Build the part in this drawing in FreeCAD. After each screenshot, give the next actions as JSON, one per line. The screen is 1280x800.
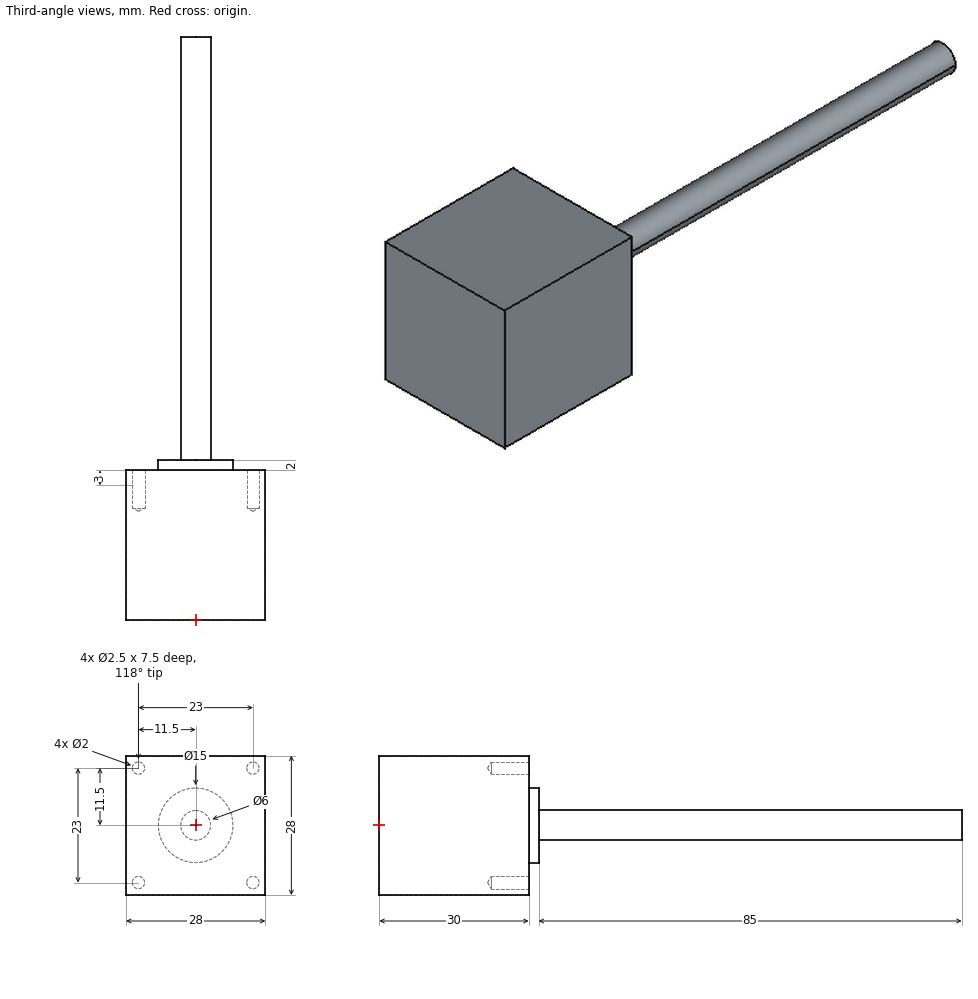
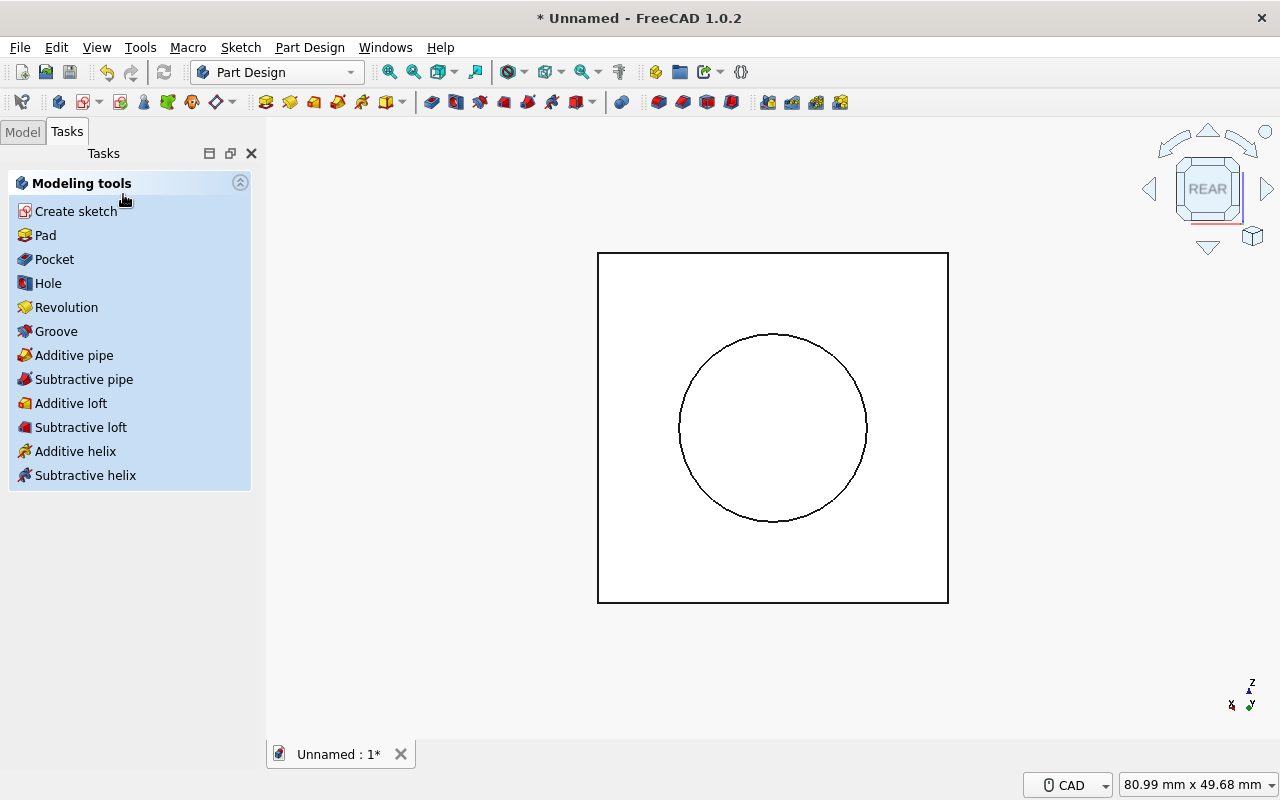
{"action": "left_click", "coordinate": [266, 102]}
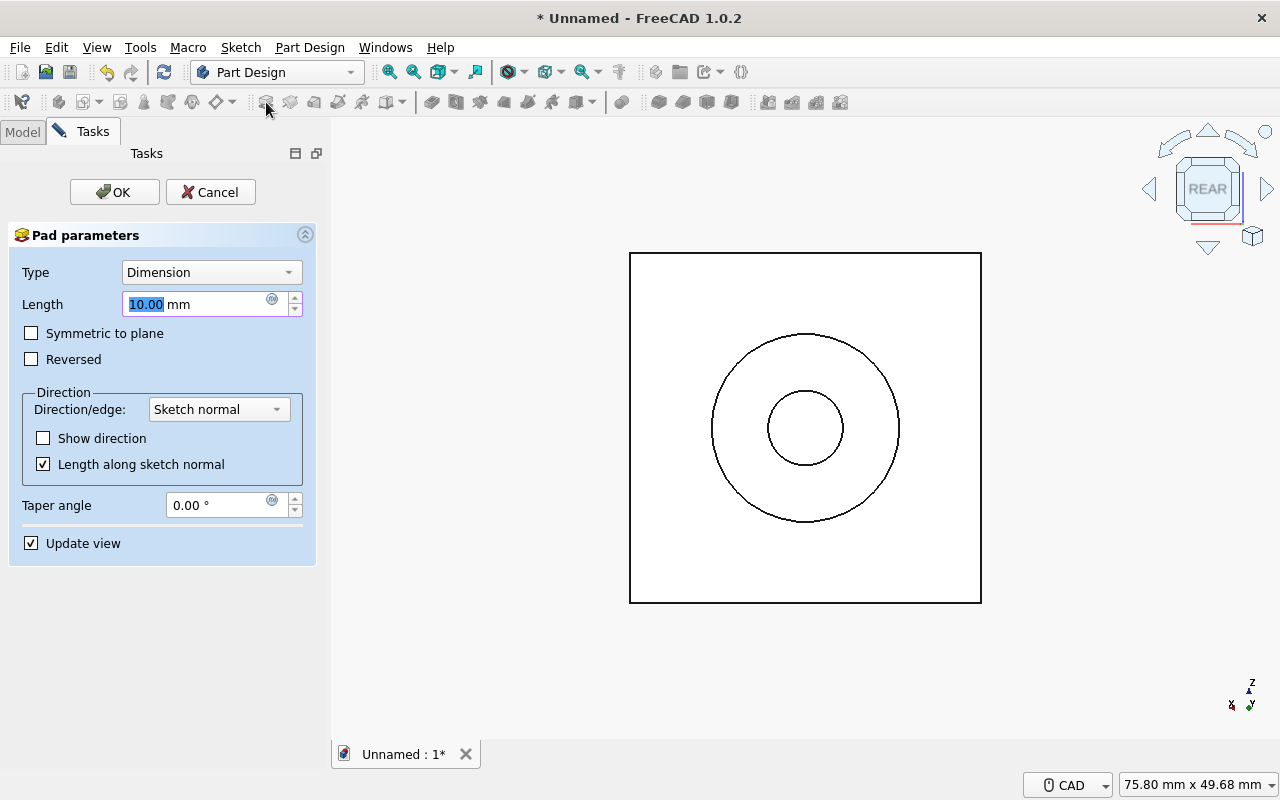
{"action": "type", "text": "85"}
{"action": "key", "text": "Tab"}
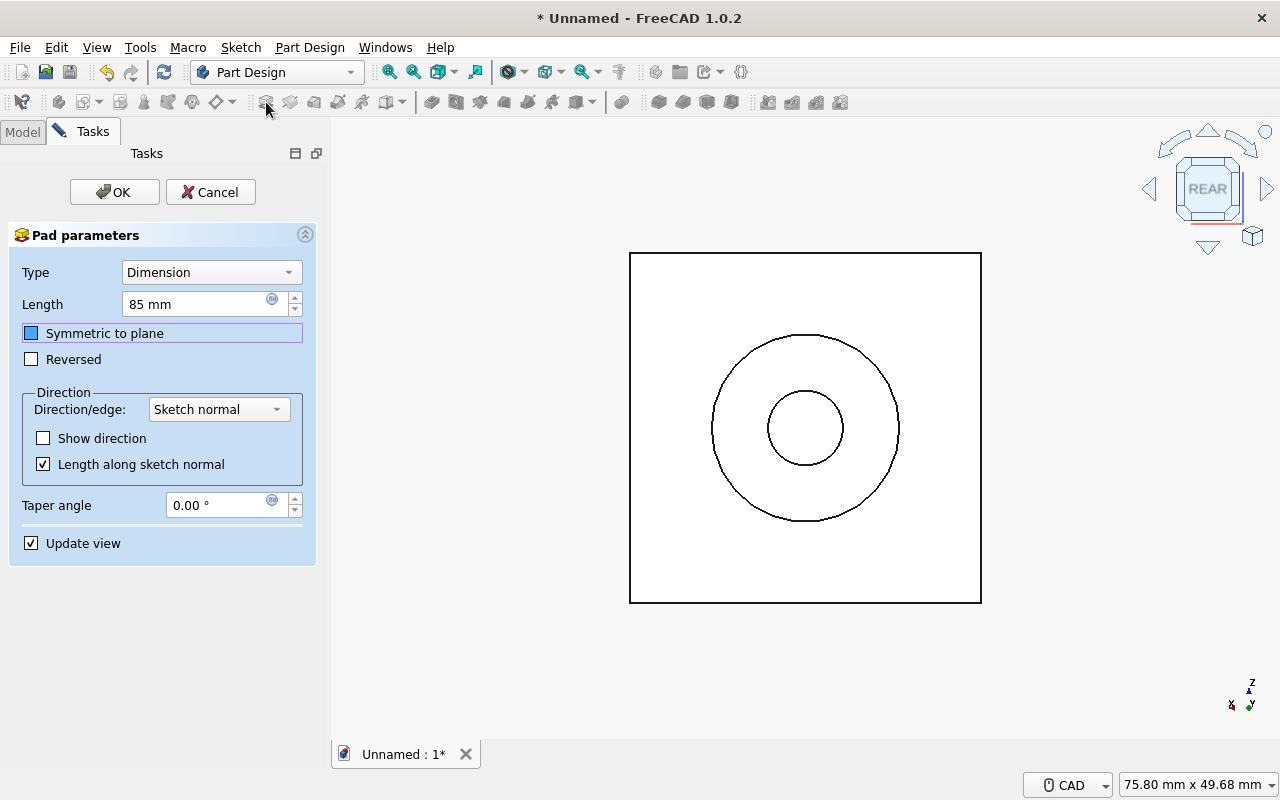
{"action": "left_click", "coordinate": [115, 192]}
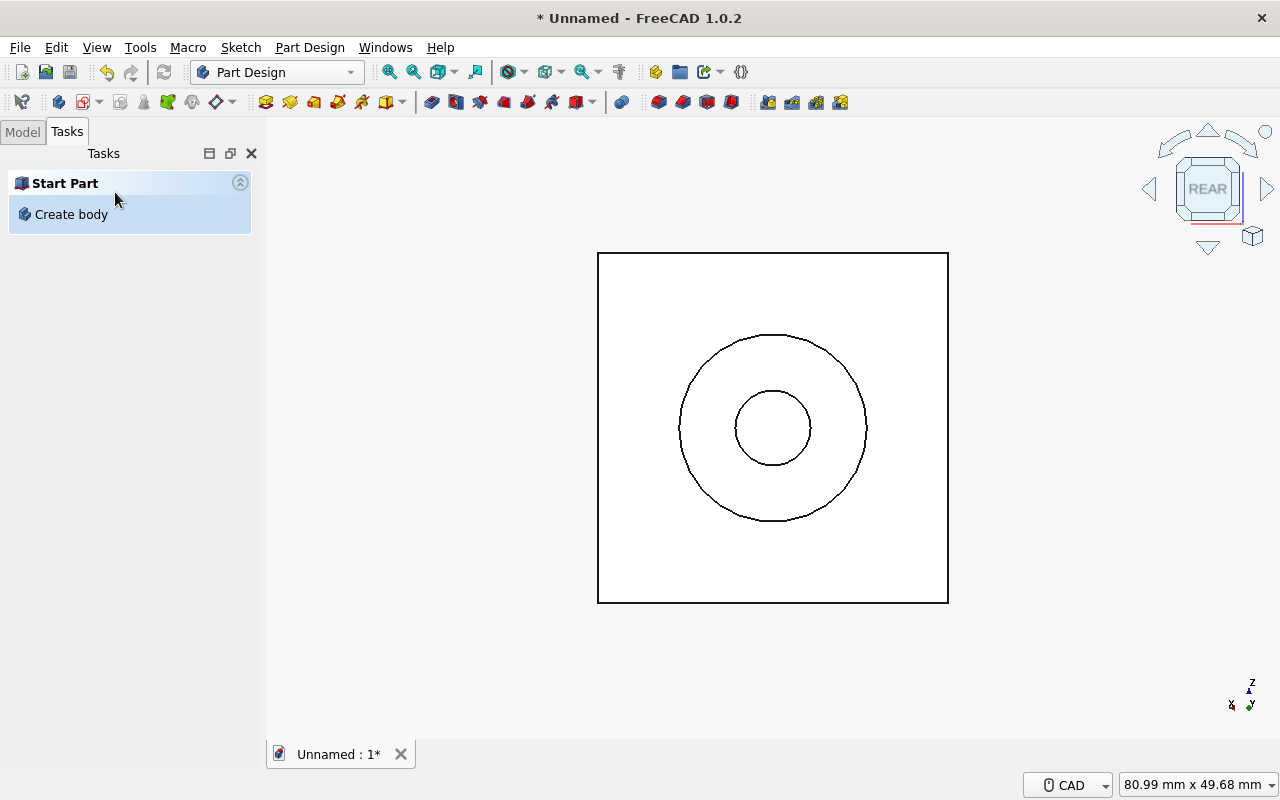
{"action": "left_click", "coordinate": [673, 527]}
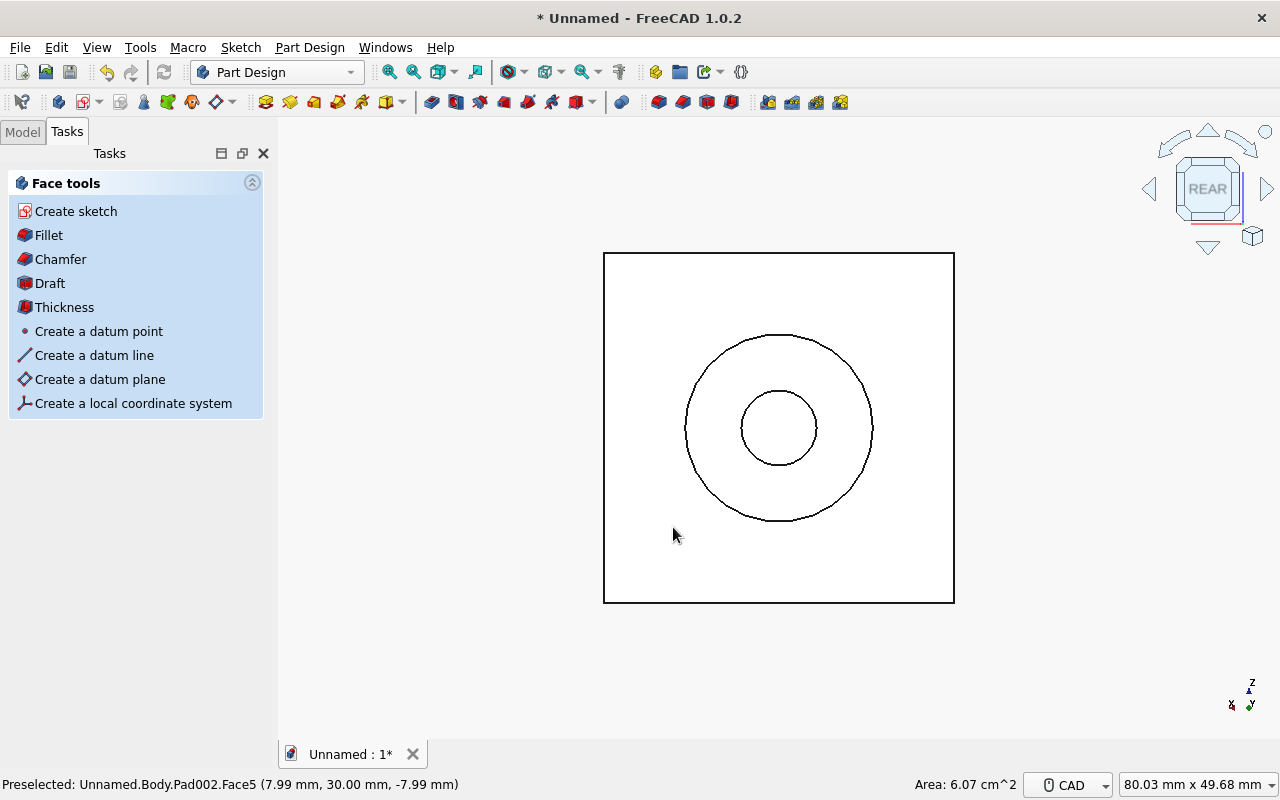
{"action": "left_click", "coordinate": [84, 102]}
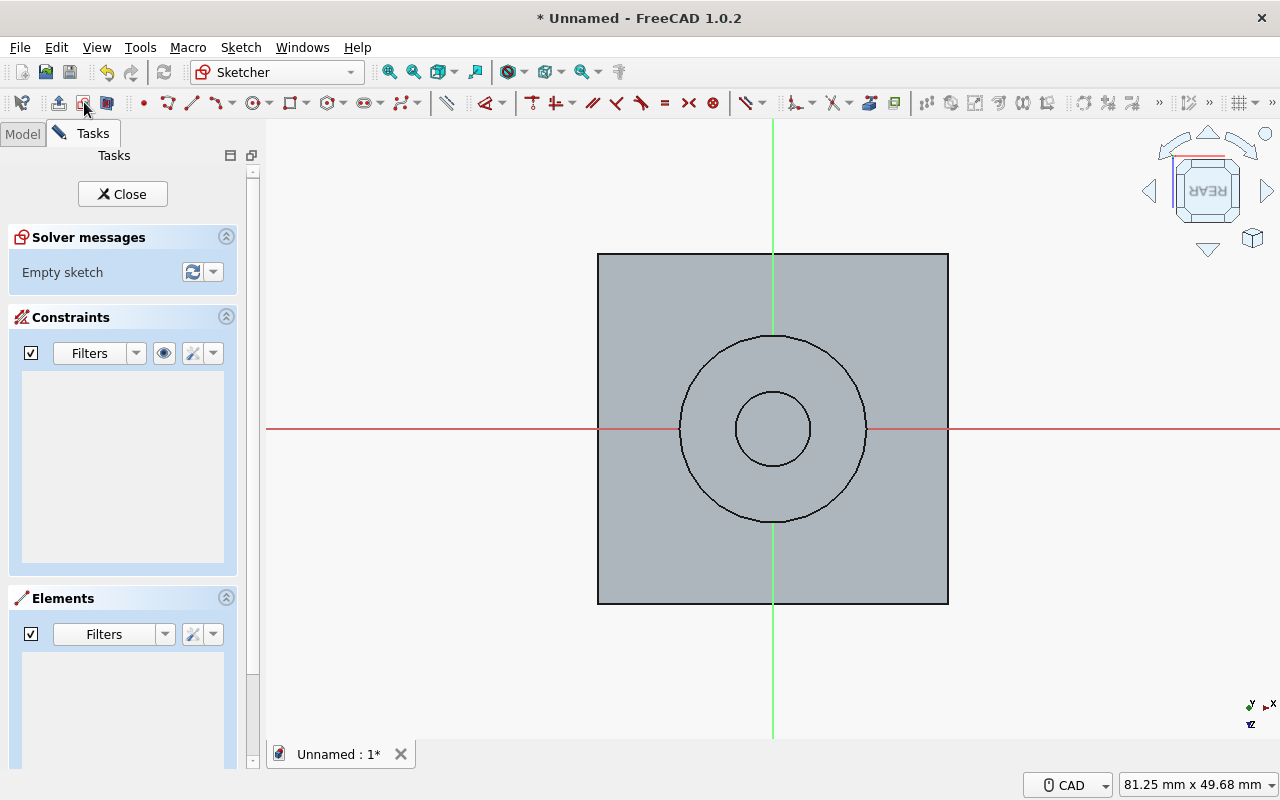
{"action": "left_click", "coordinate": [254, 104]}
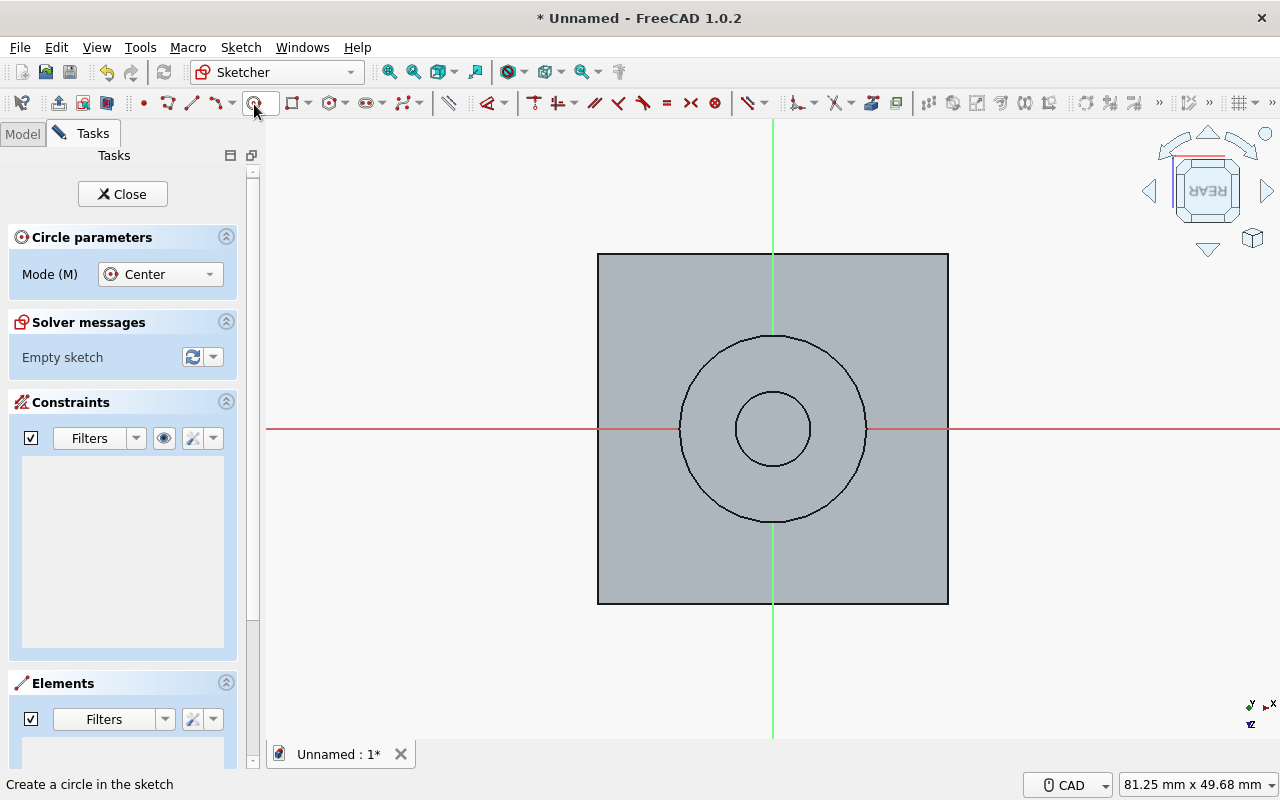
{"action": "scroll", "coordinate": [629, 573], "scroll_direction": "up", "scroll_amount": 3}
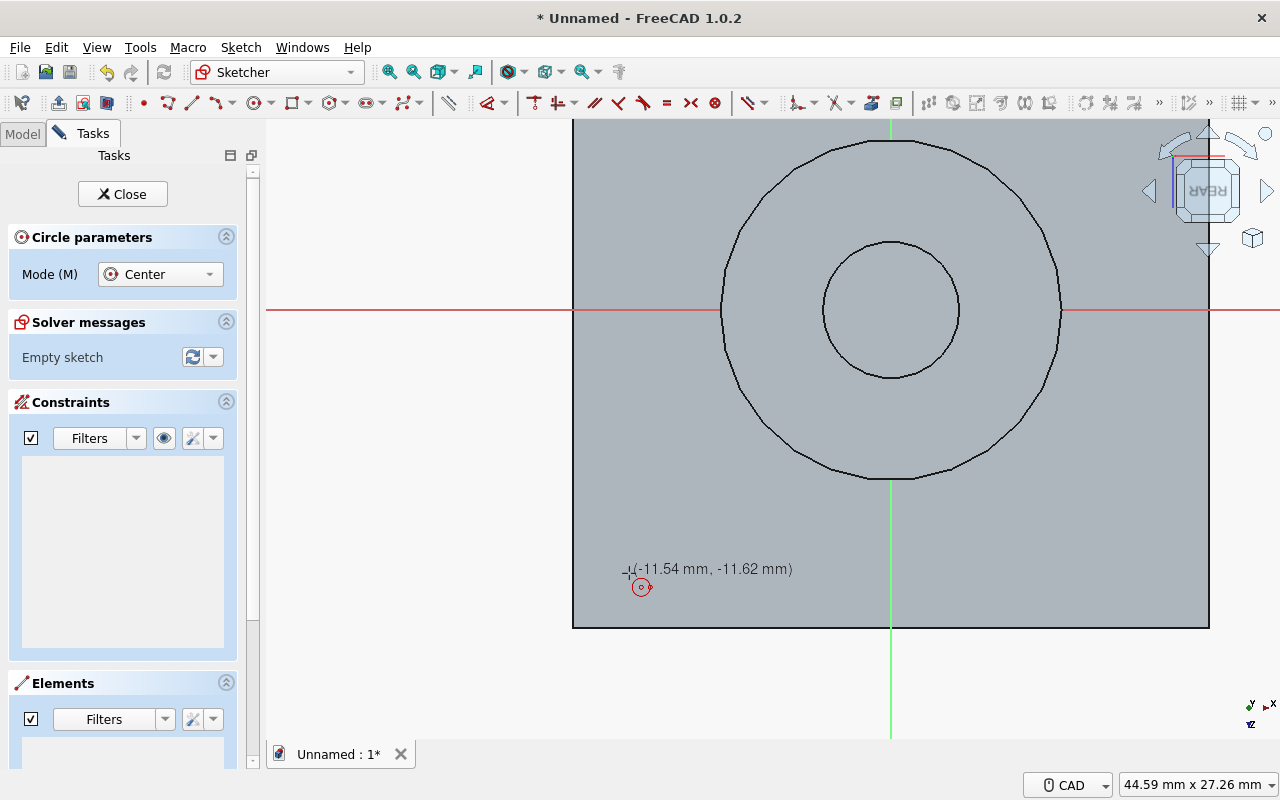
{"action": "left_click", "coordinate": [630, 572]}
{"action": "left_click", "coordinate": [646, 555]}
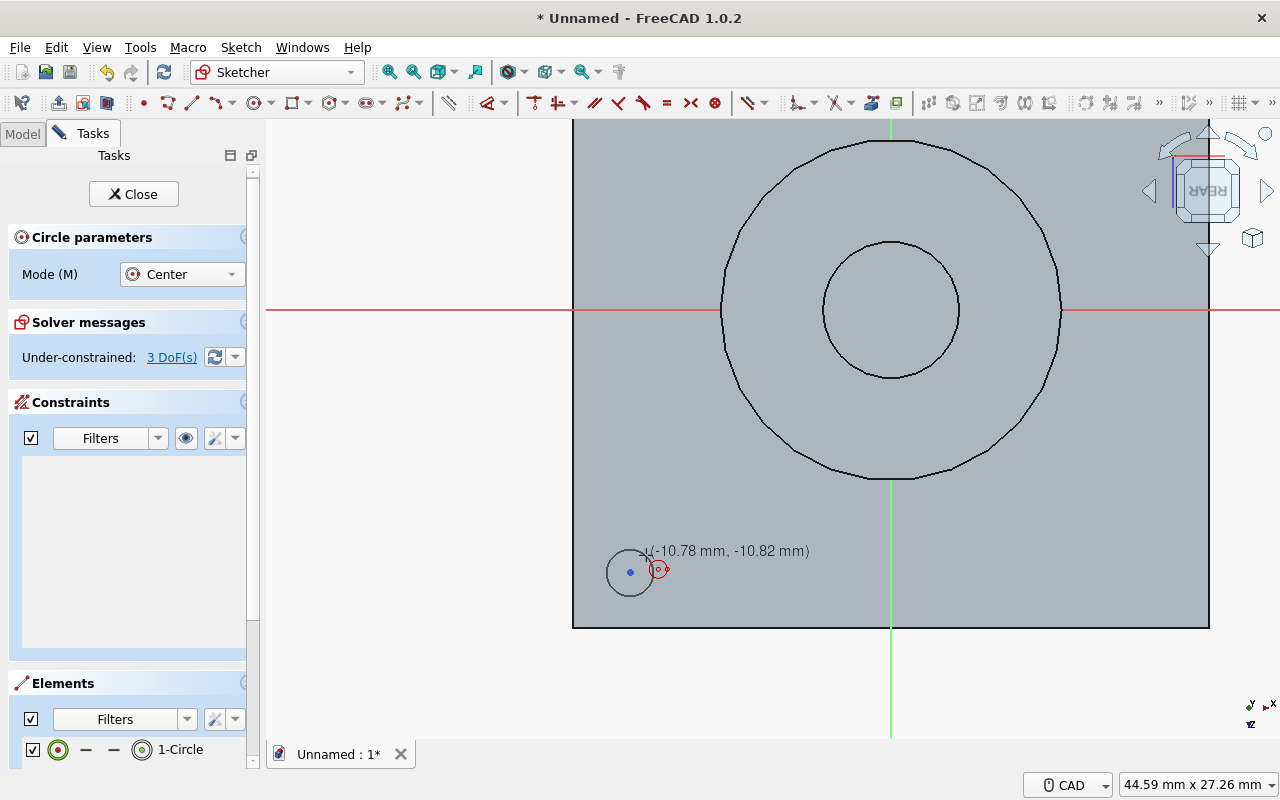
{"action": "scroll", "coordinate": [325, 671], "scroll_direction": "down", "scroll_amount": 2}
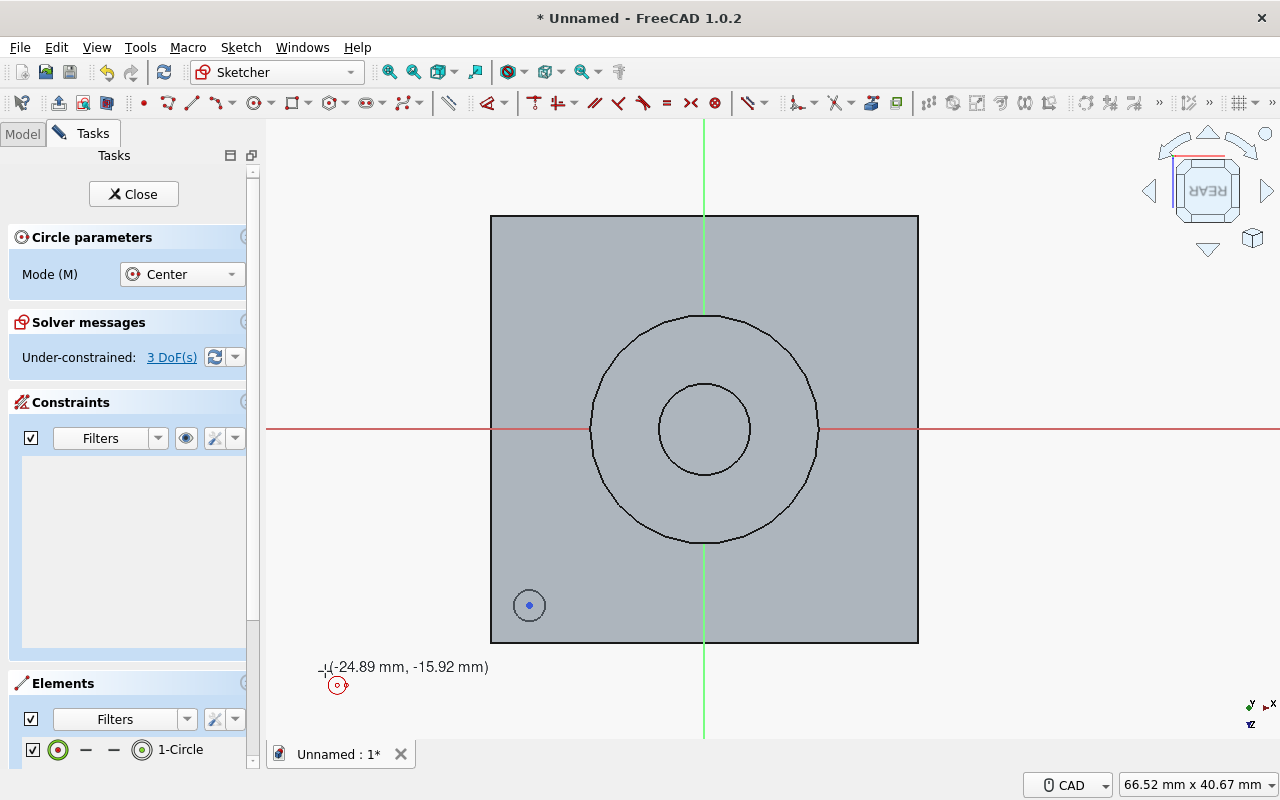
{"action": "scroll", "coordinate": [880, 605], "scroll_direction": "up", "scroll_amount": 2}